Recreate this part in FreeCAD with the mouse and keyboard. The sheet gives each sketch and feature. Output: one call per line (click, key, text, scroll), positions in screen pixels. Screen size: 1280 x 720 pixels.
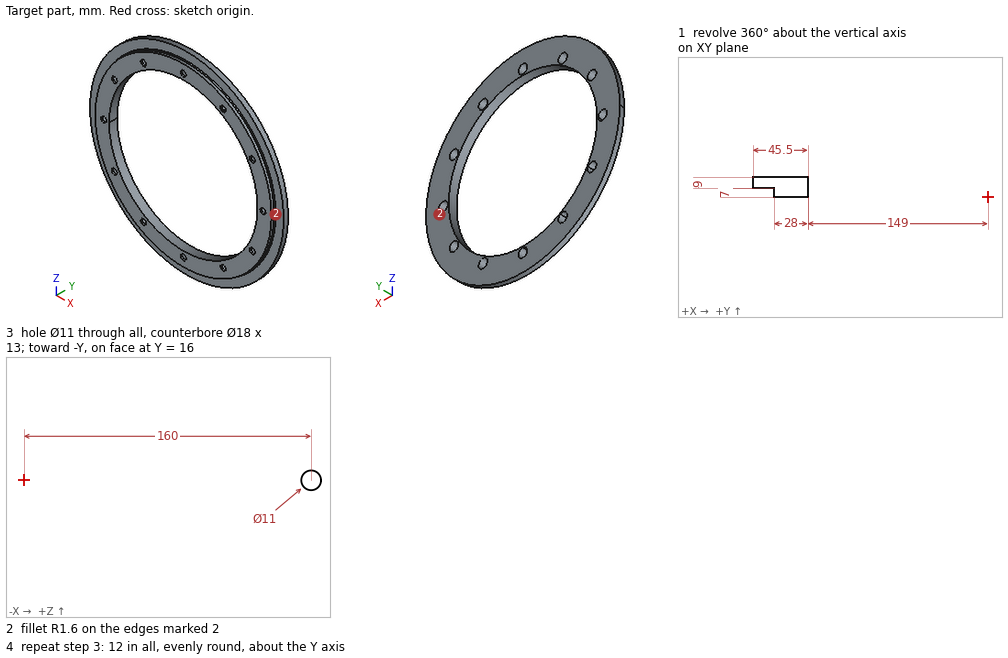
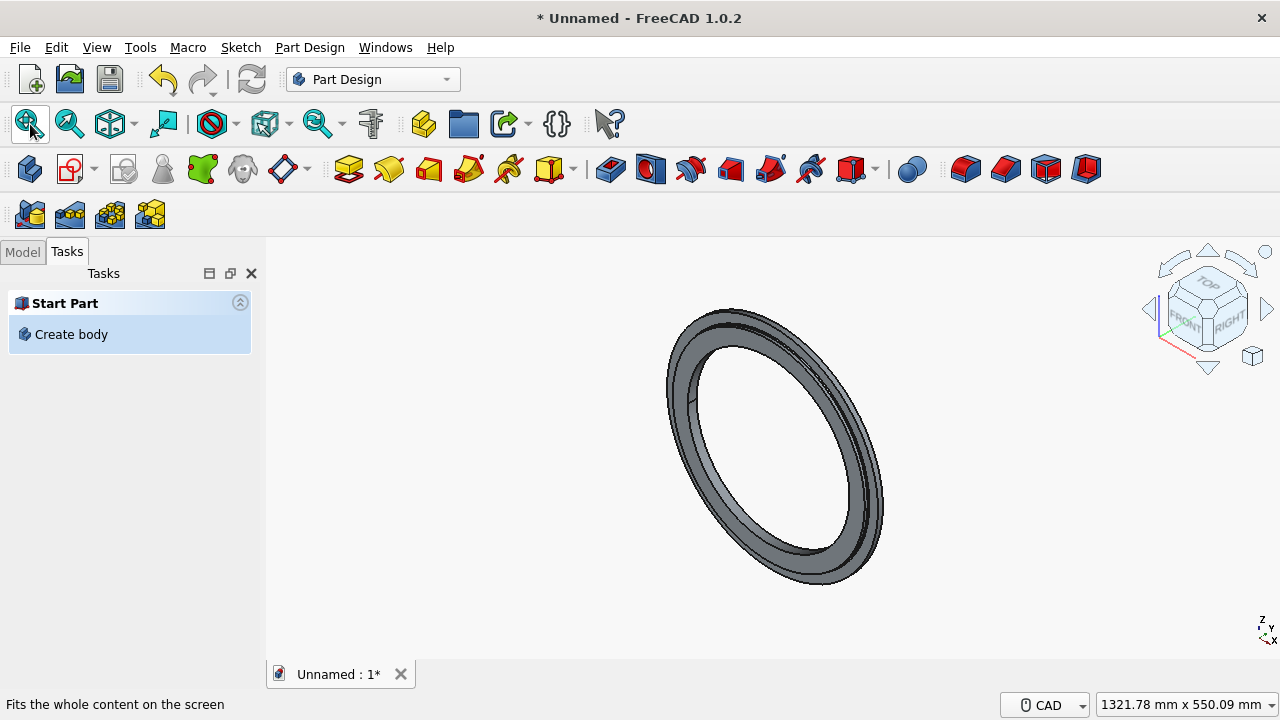
key(4)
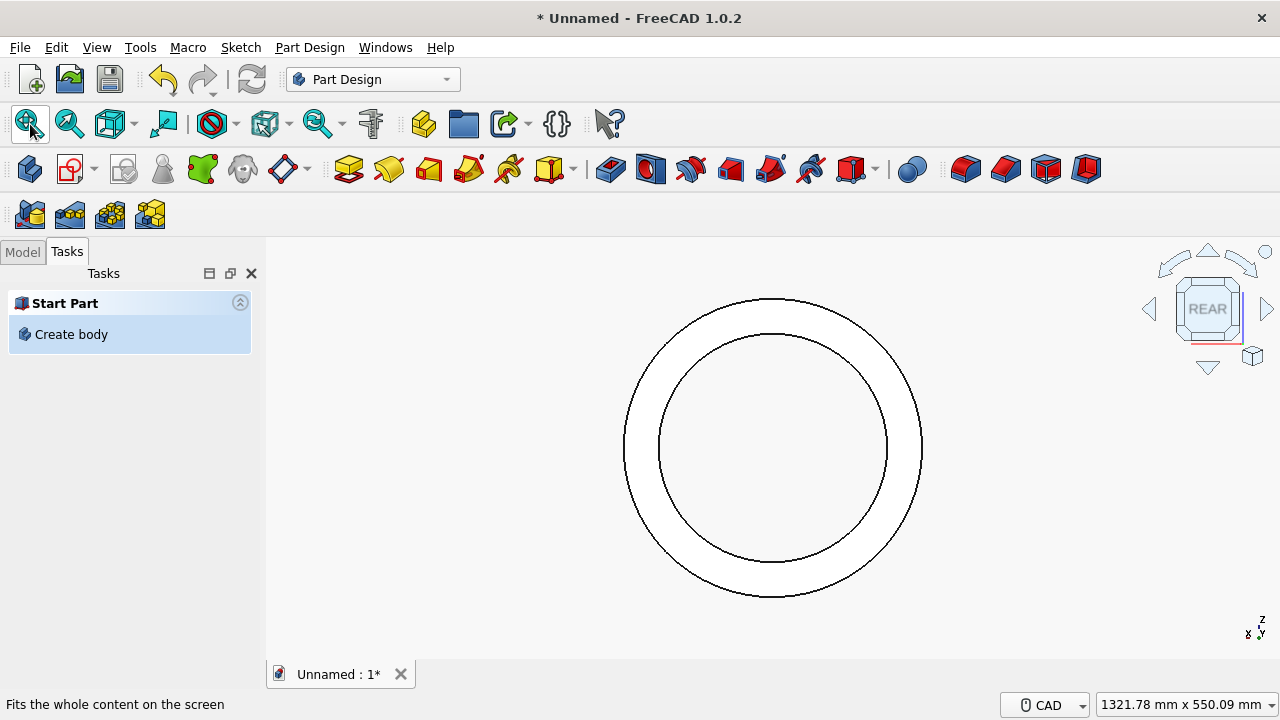
click(645, 490)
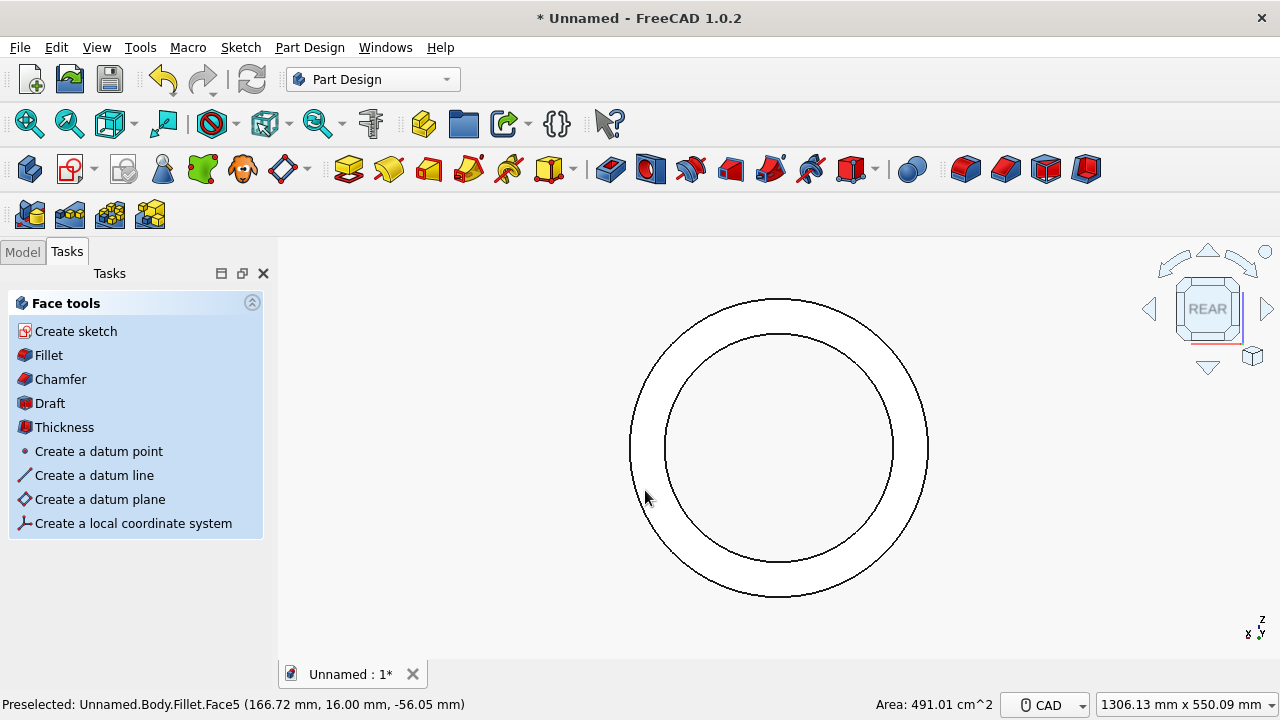
click(70, 170)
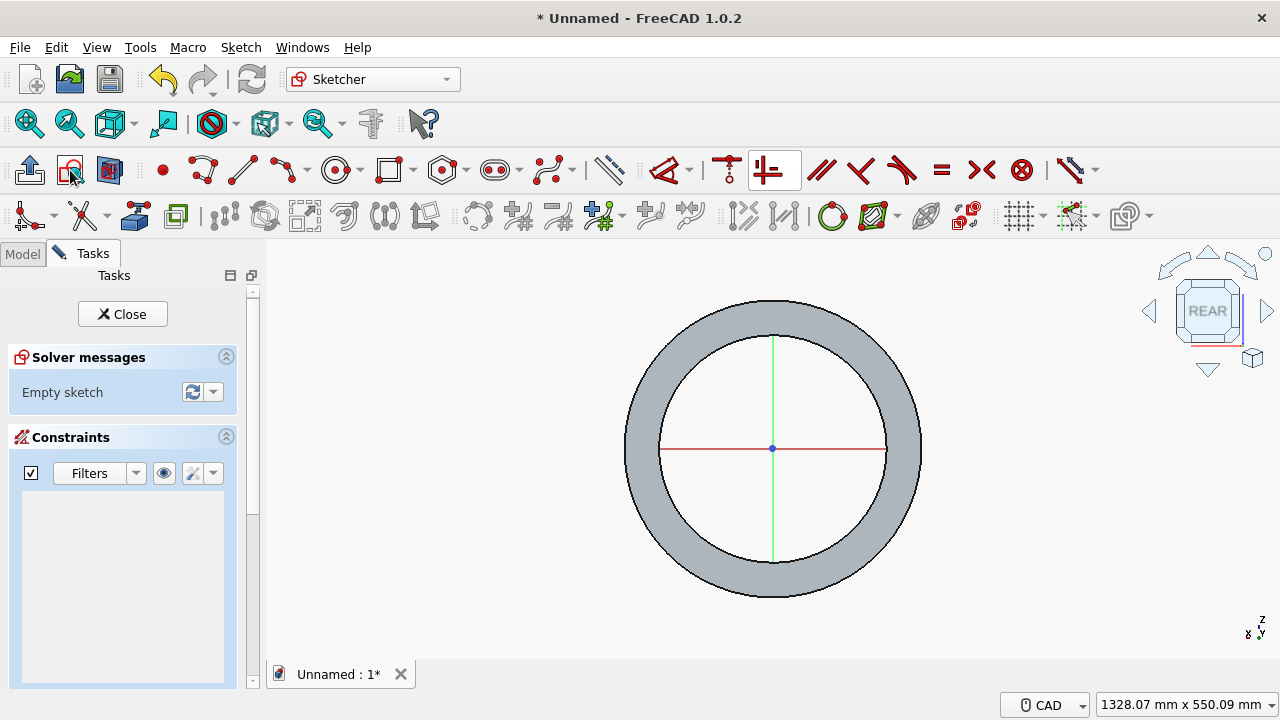
scroll(905, 449, up, 15)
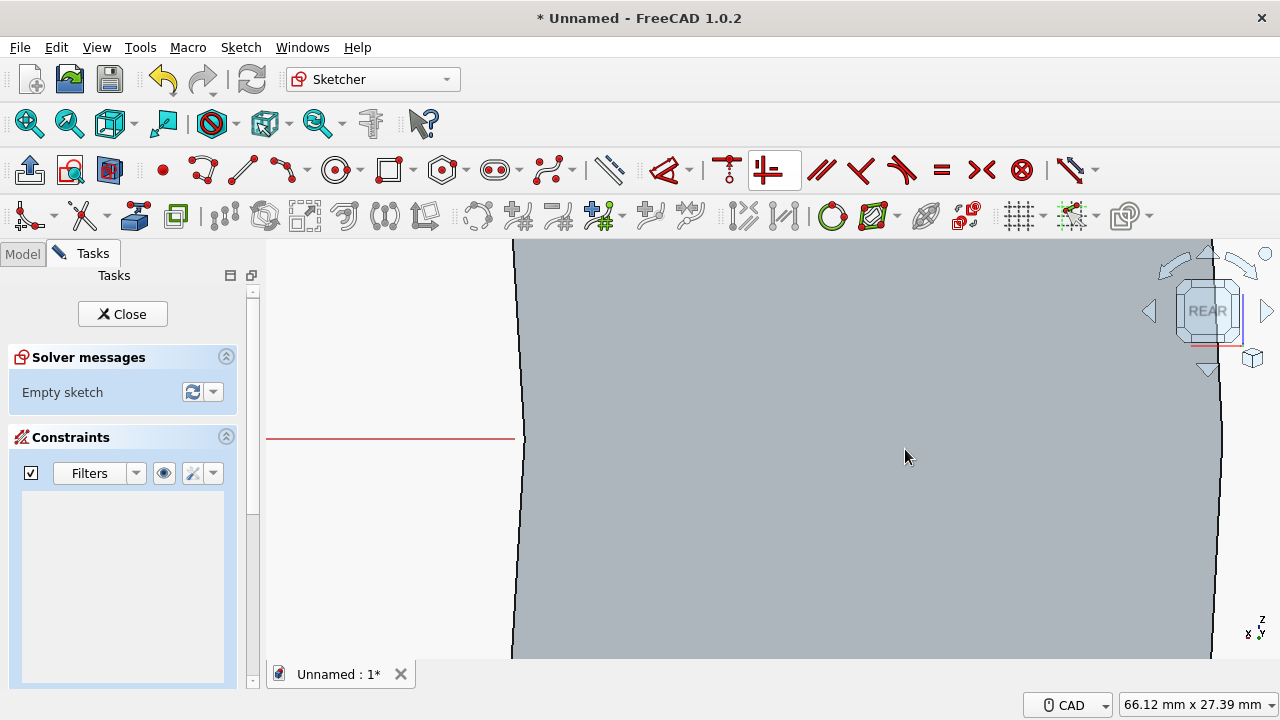
scroll(671, 420, up, 2)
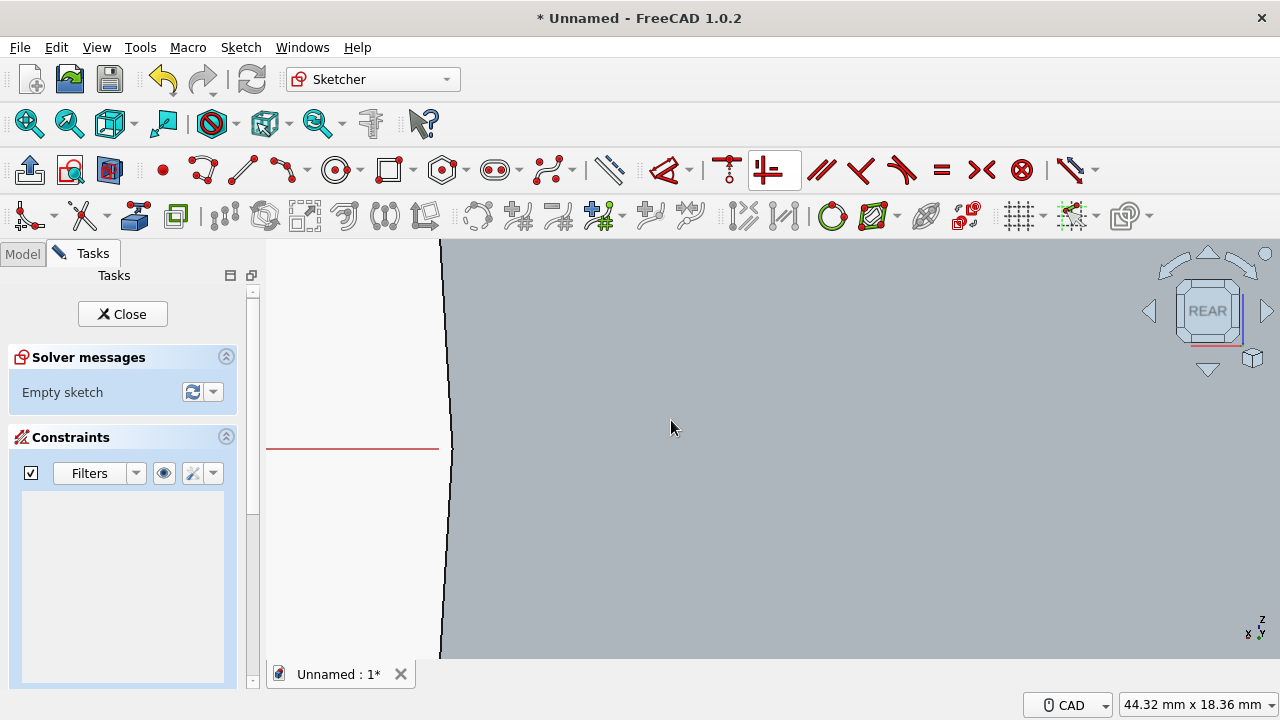
click(336, 170)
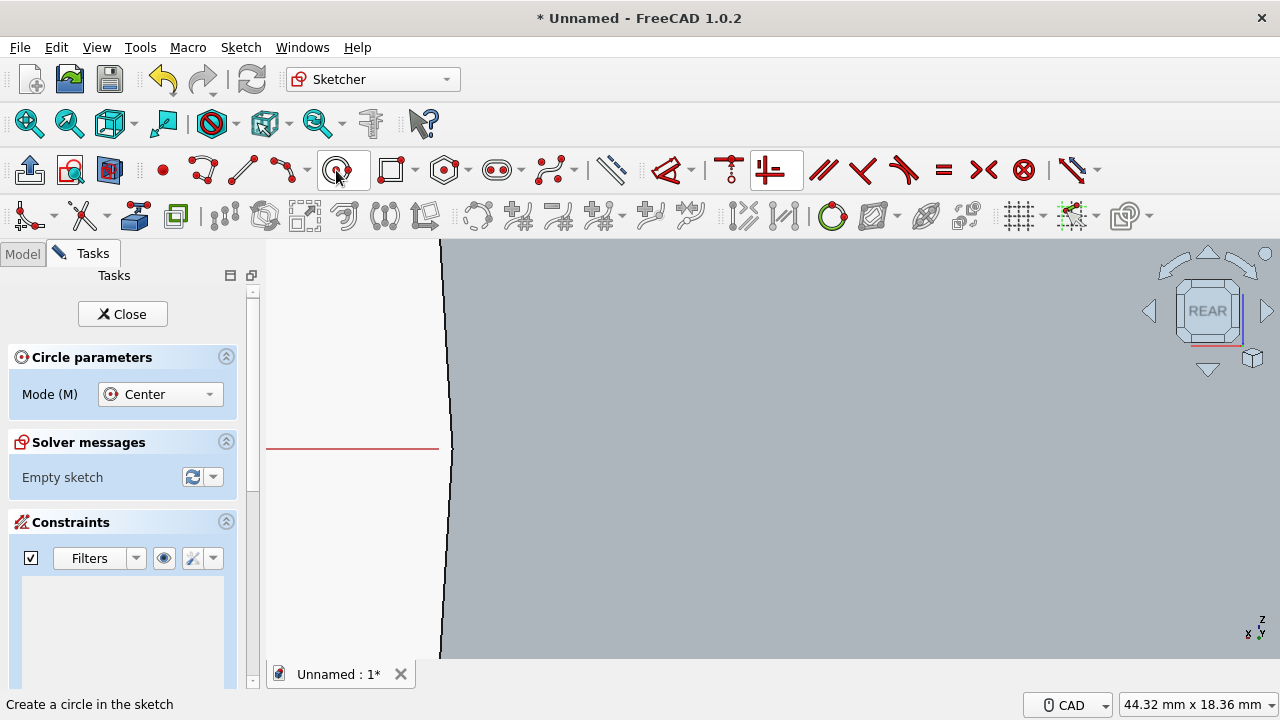
click(704, 449)
click(793, 360)
key(Escape)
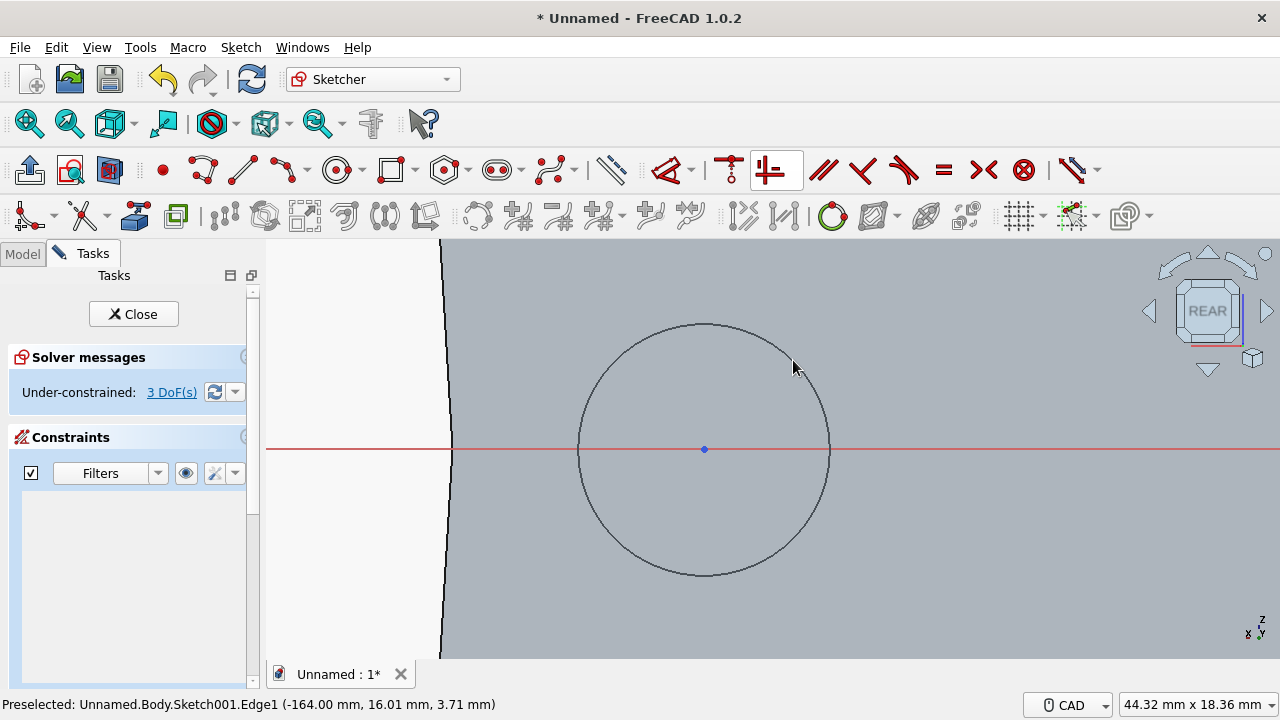
click(704, 450)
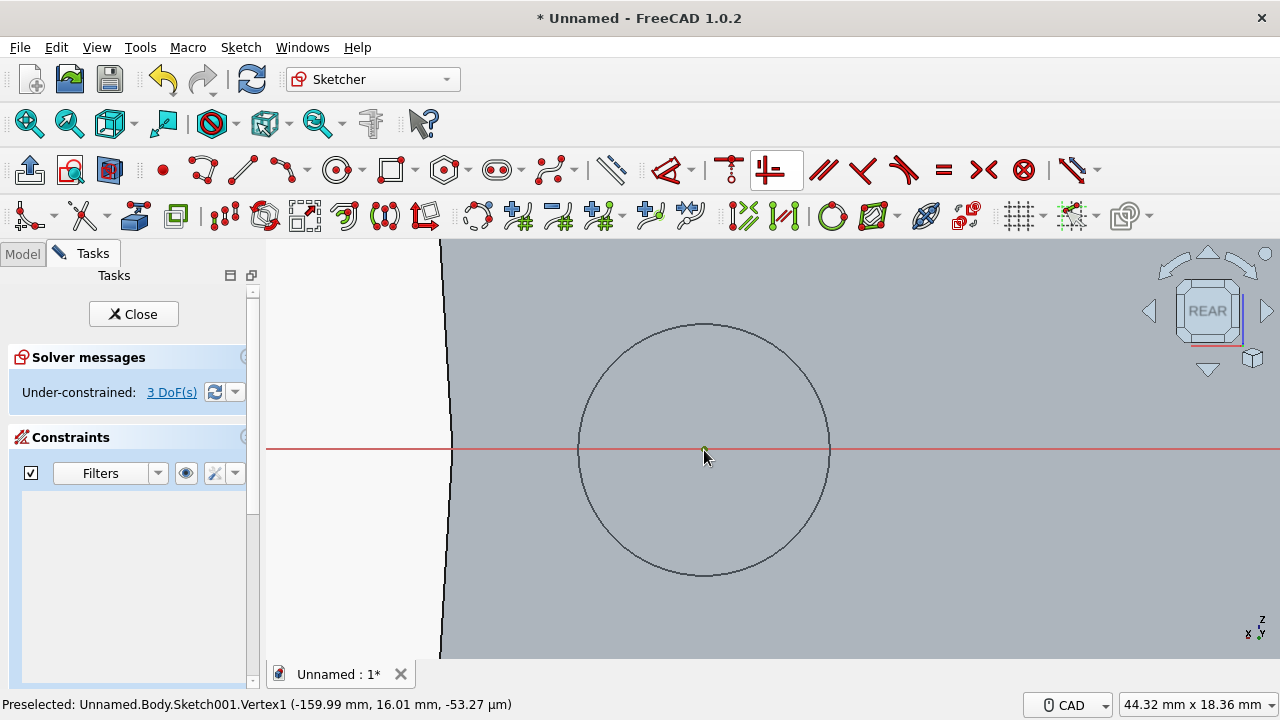
click(353, 449)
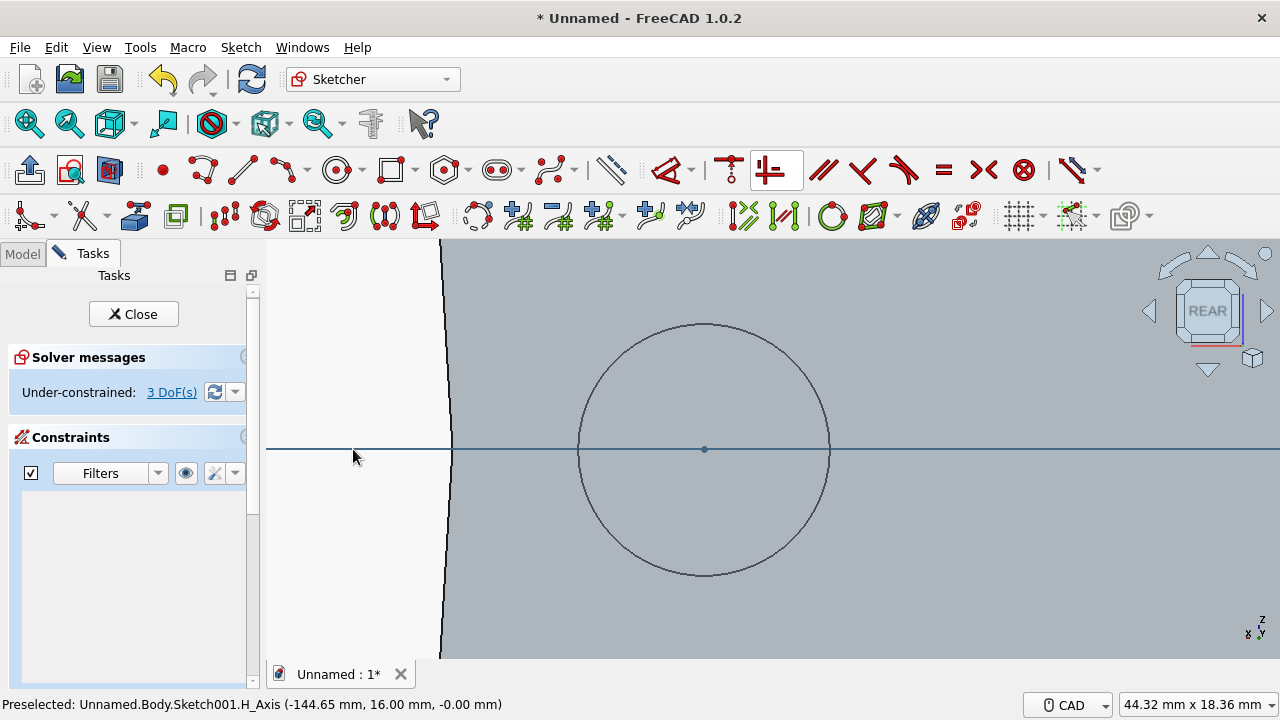
click(730, 170)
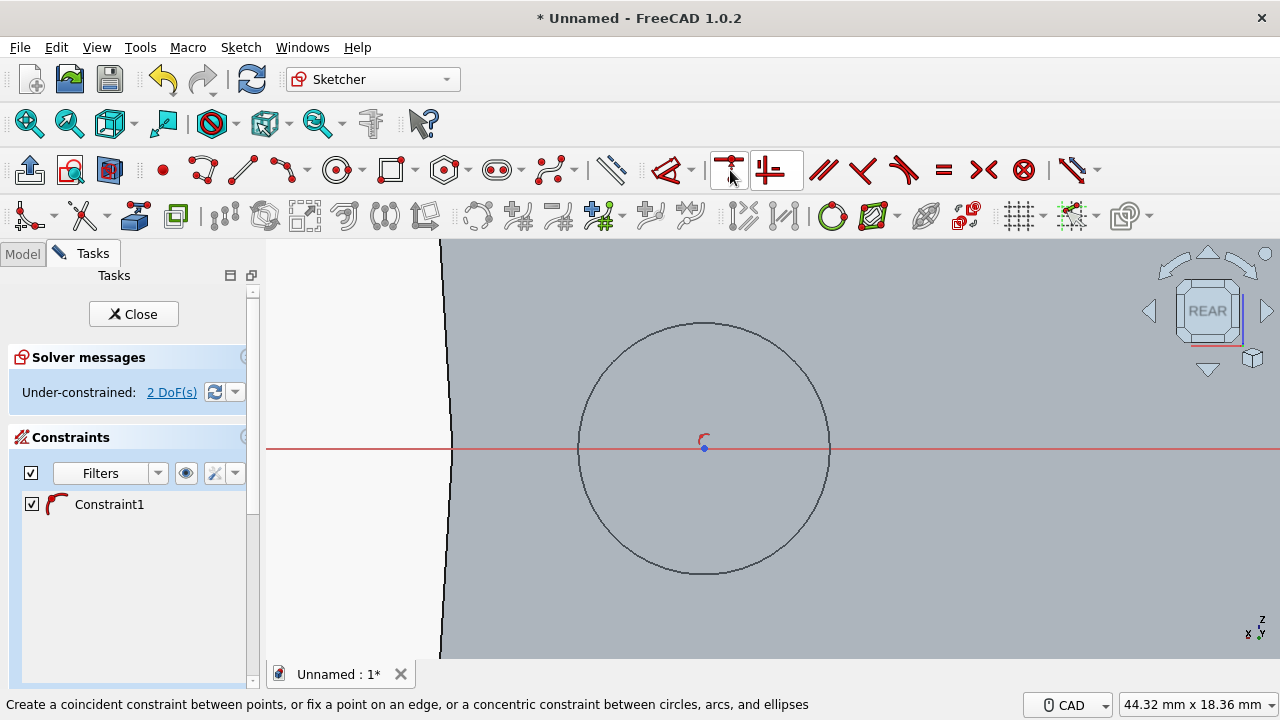
click(666, 170)